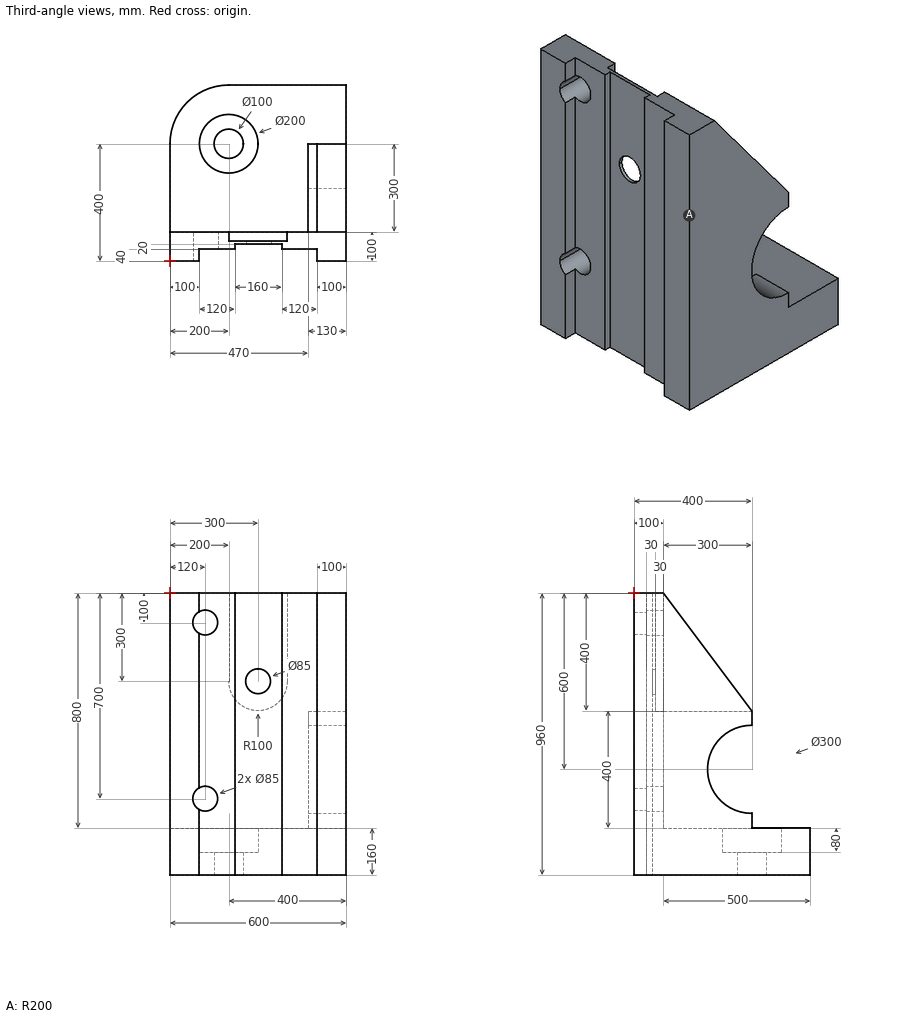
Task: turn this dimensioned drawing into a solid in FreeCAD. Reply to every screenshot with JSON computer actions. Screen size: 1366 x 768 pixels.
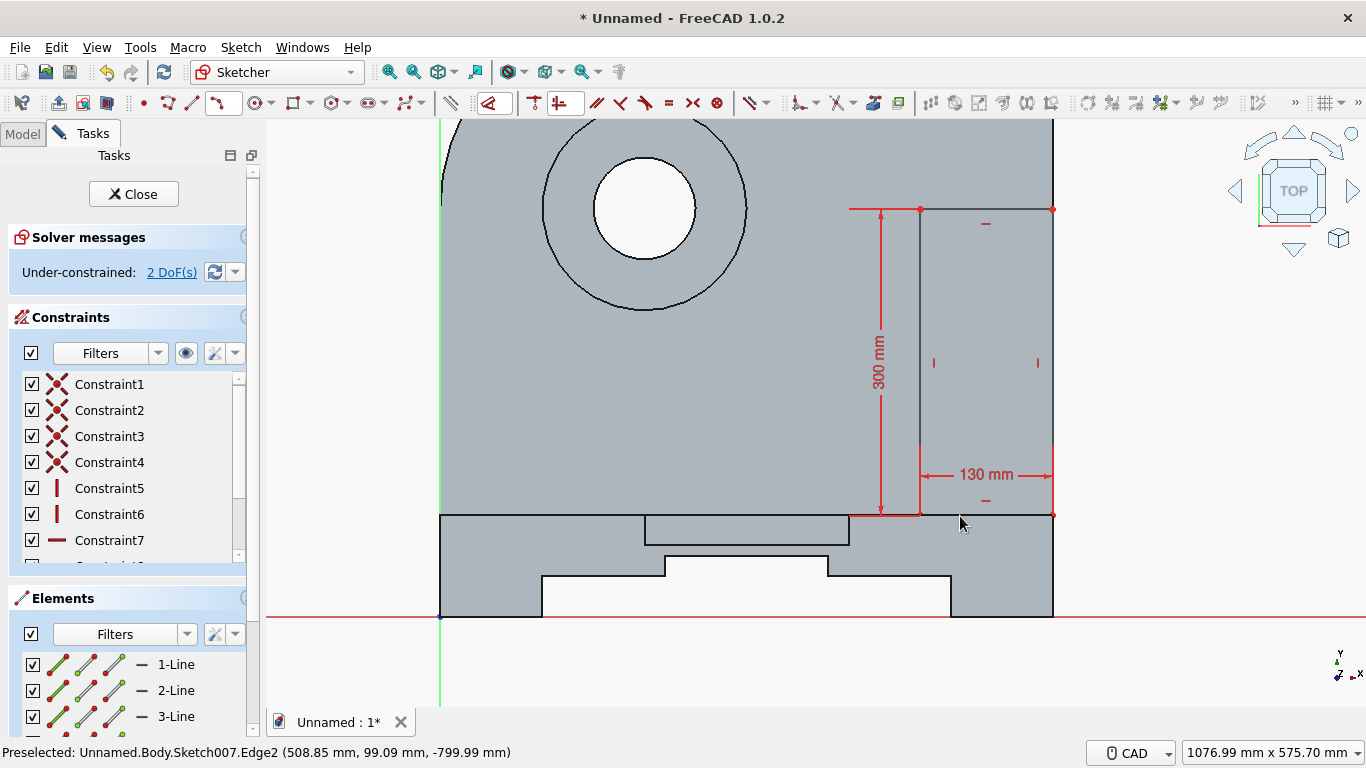
{"action": "left_click", "coordinate": [920, 209]}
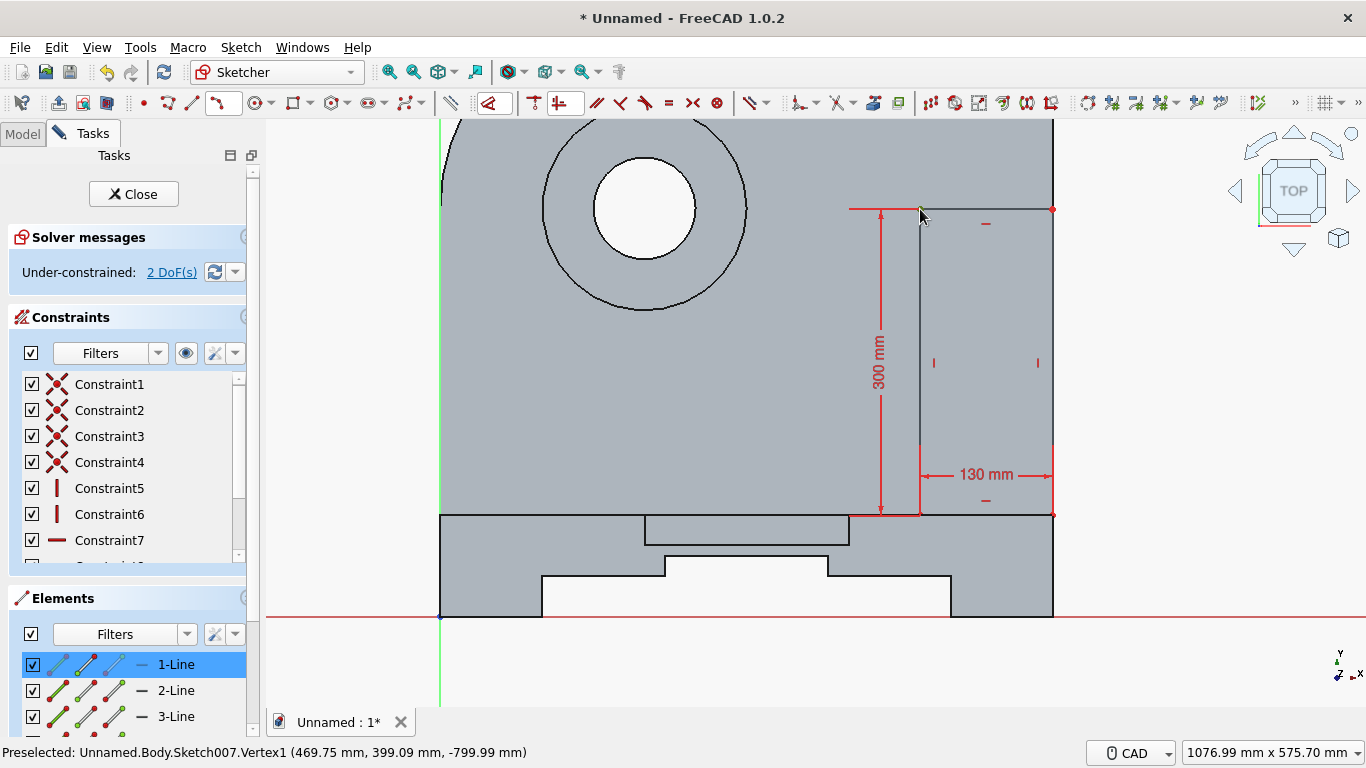
{"action": "left_click", "coordinate": [506, 104]}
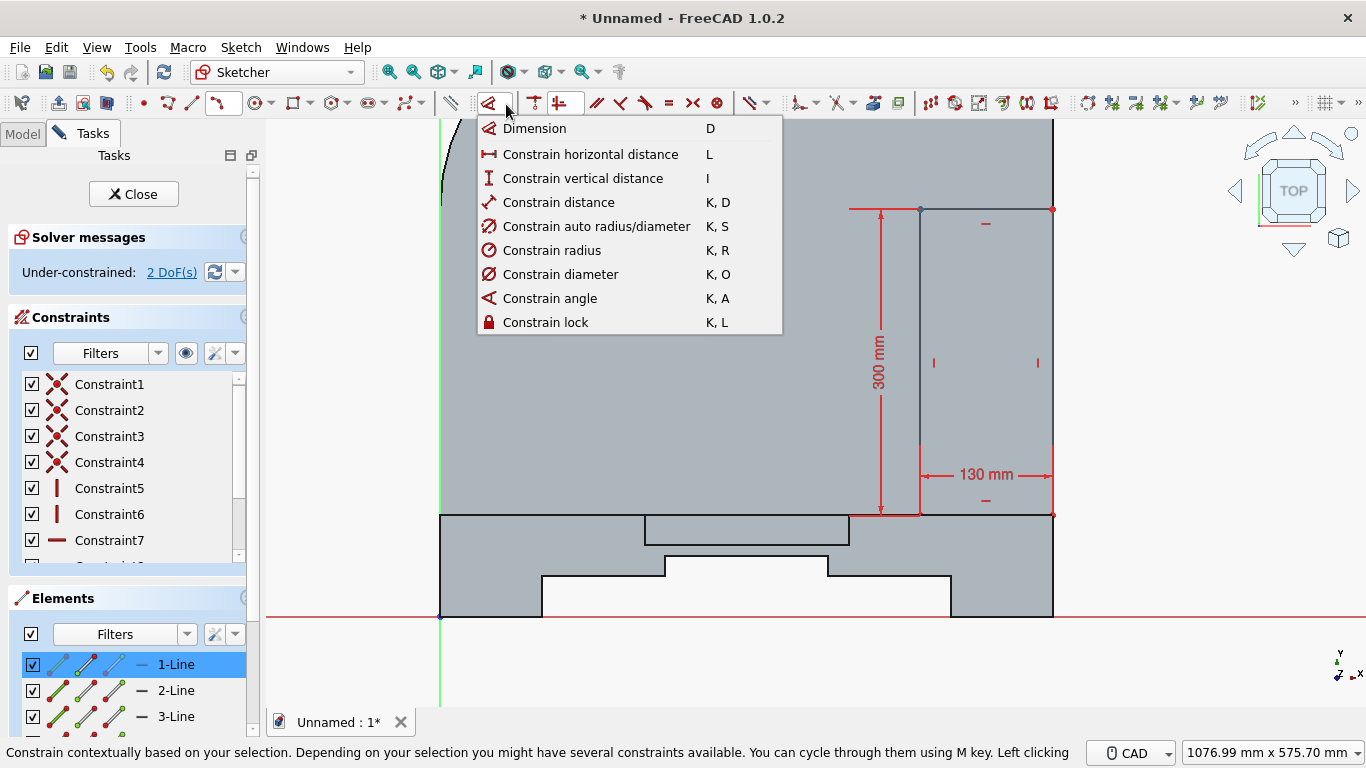
{"action": "left_click", "coordinate": [630, 154]}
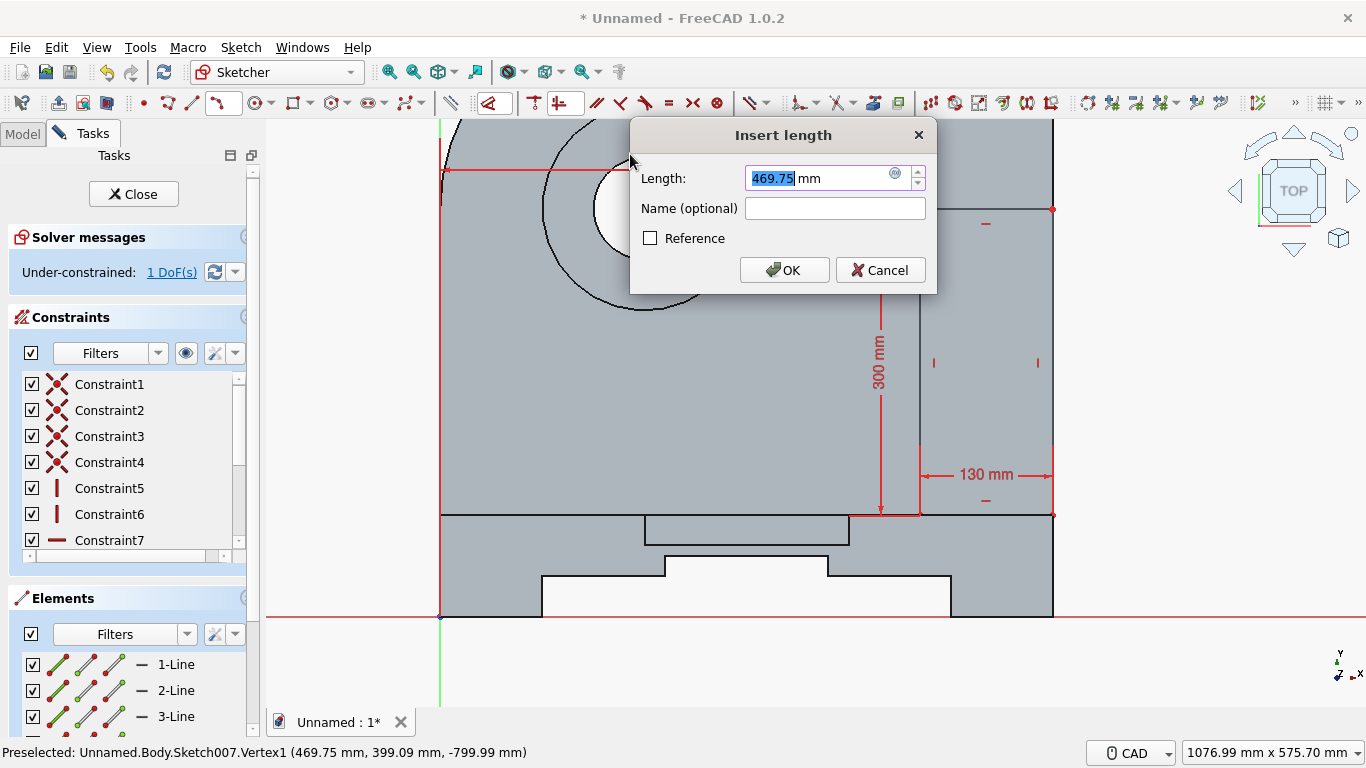
{"action": "type", "text": "470"}
{"action": "key", "text": "Return"}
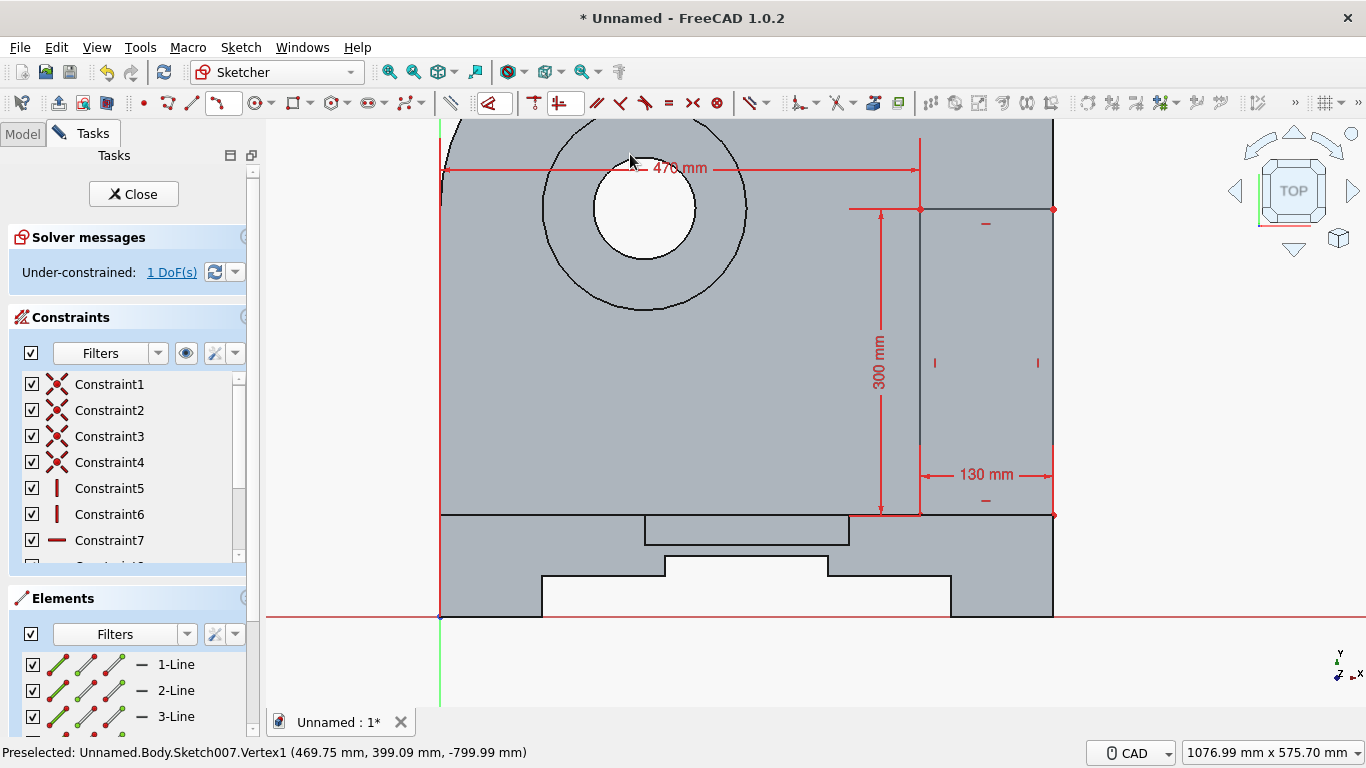
{"action": "left_click", "coordinate": [920, 209]}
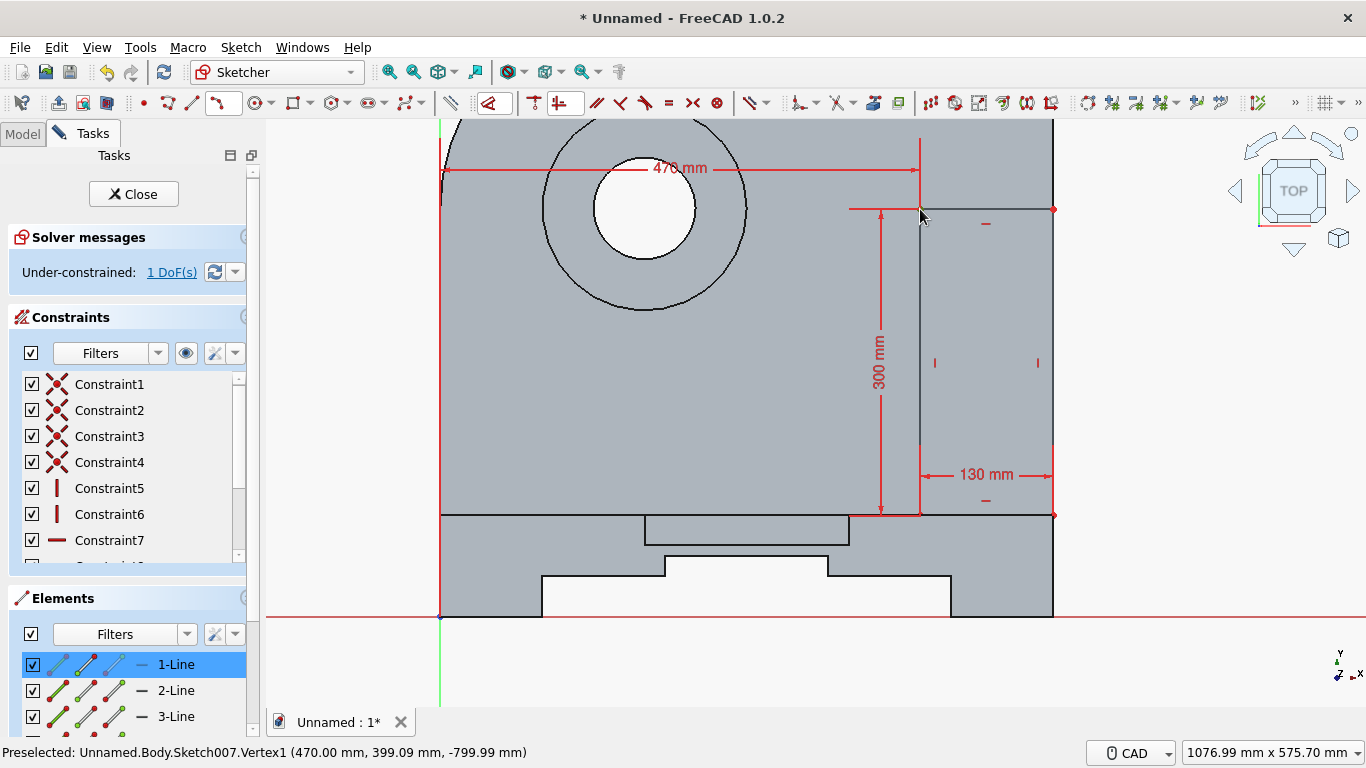
{"action": "left_click", "coordinate": [506, 104]}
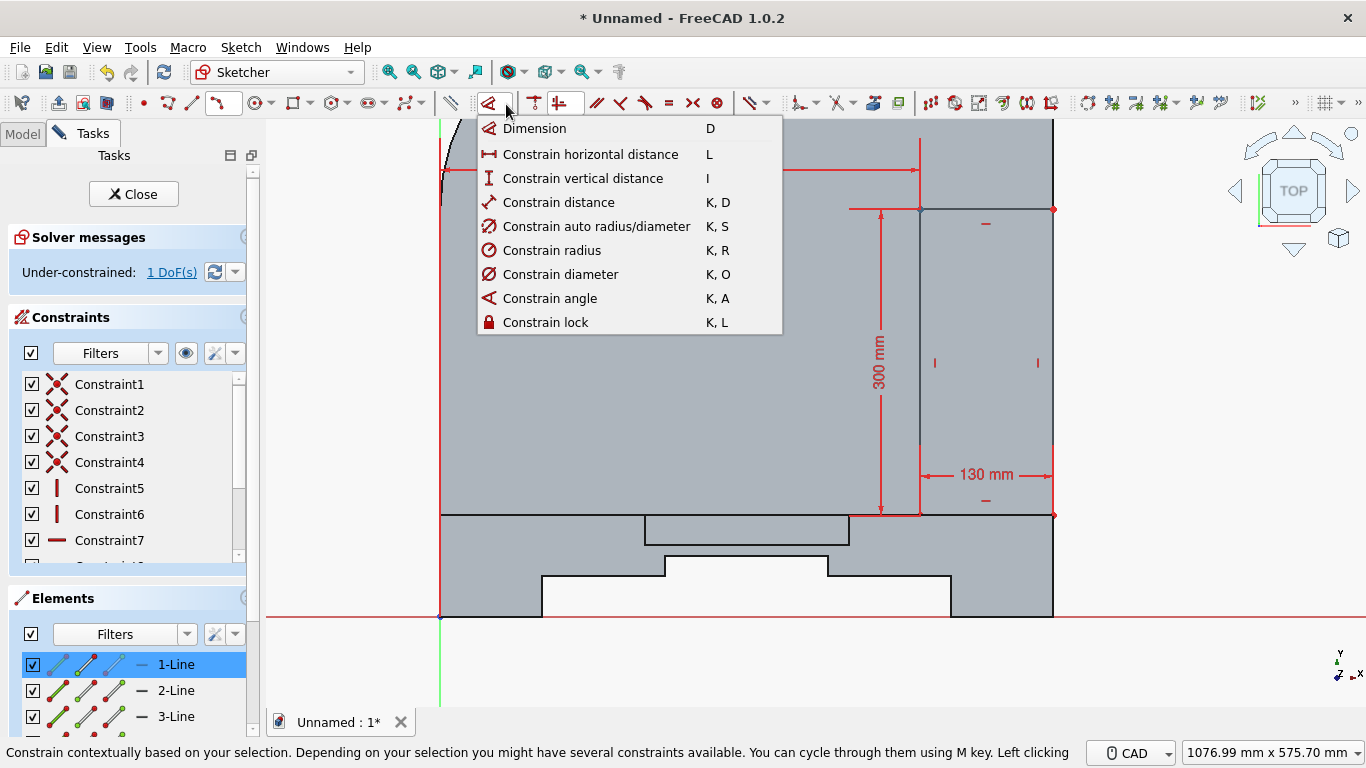
{"action": "left_click", "coordinate": [630, 178]}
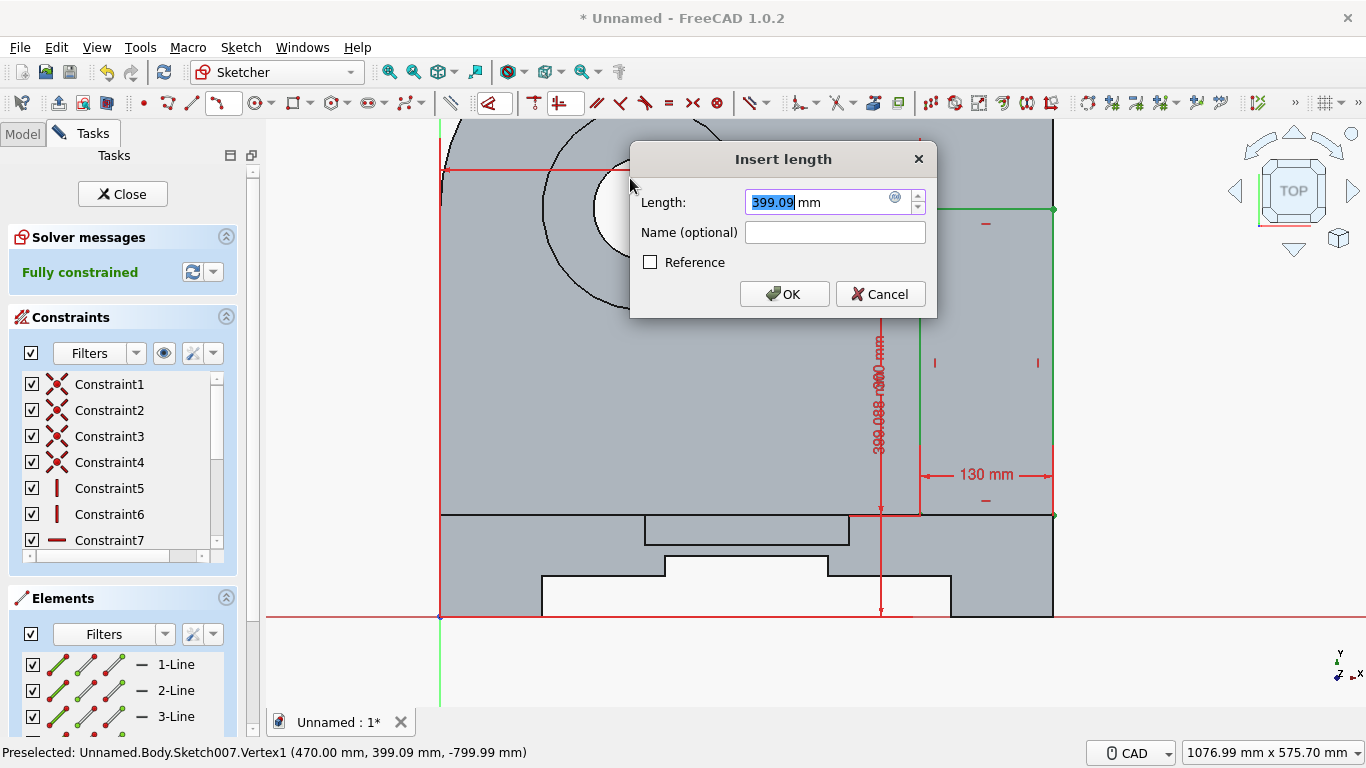
{"action": "type", "text": "400"}
{"action": "key", "text": "Return"}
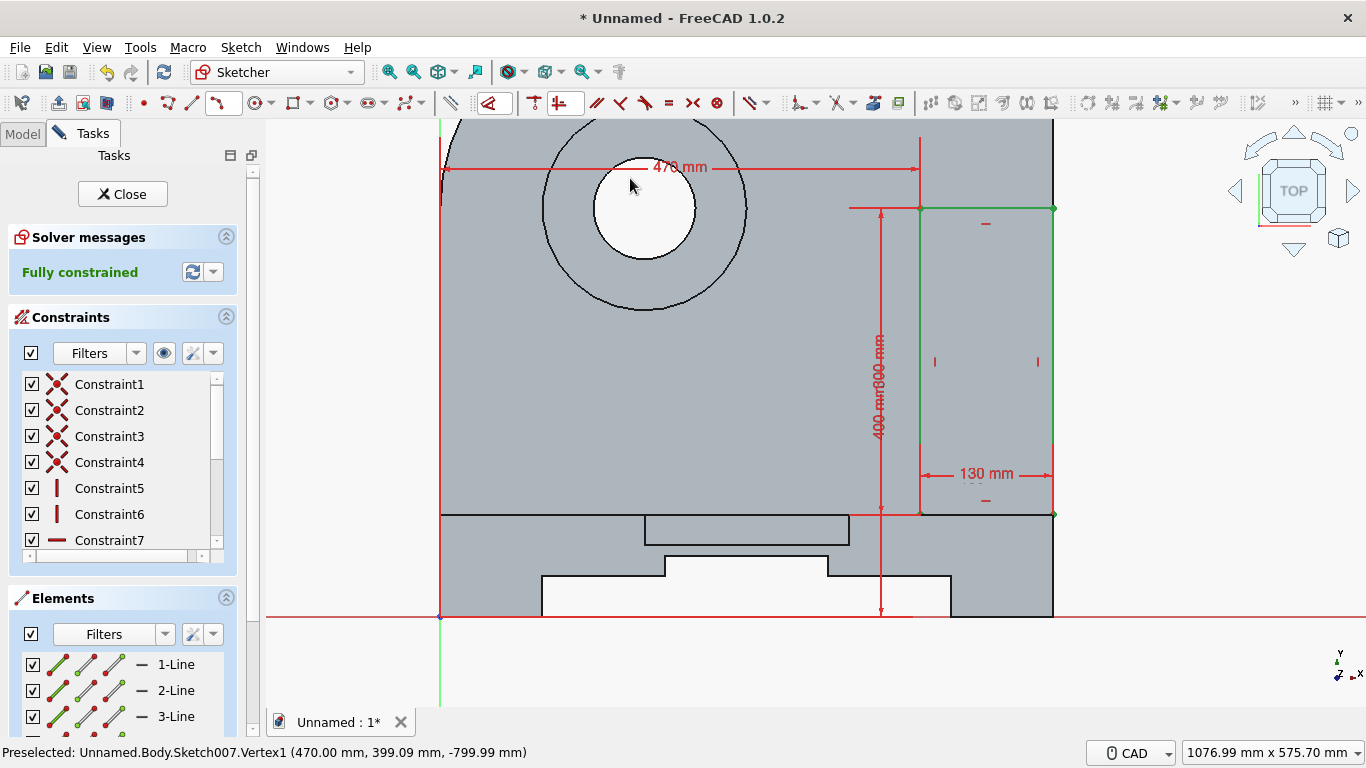
{"action": "left_click", "coordinate": [123, 194]}